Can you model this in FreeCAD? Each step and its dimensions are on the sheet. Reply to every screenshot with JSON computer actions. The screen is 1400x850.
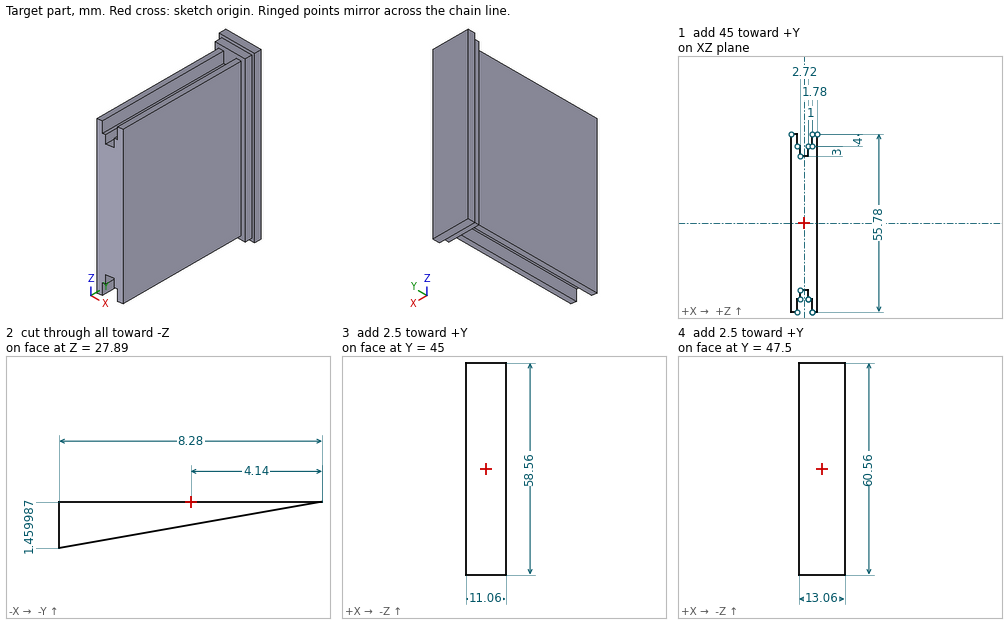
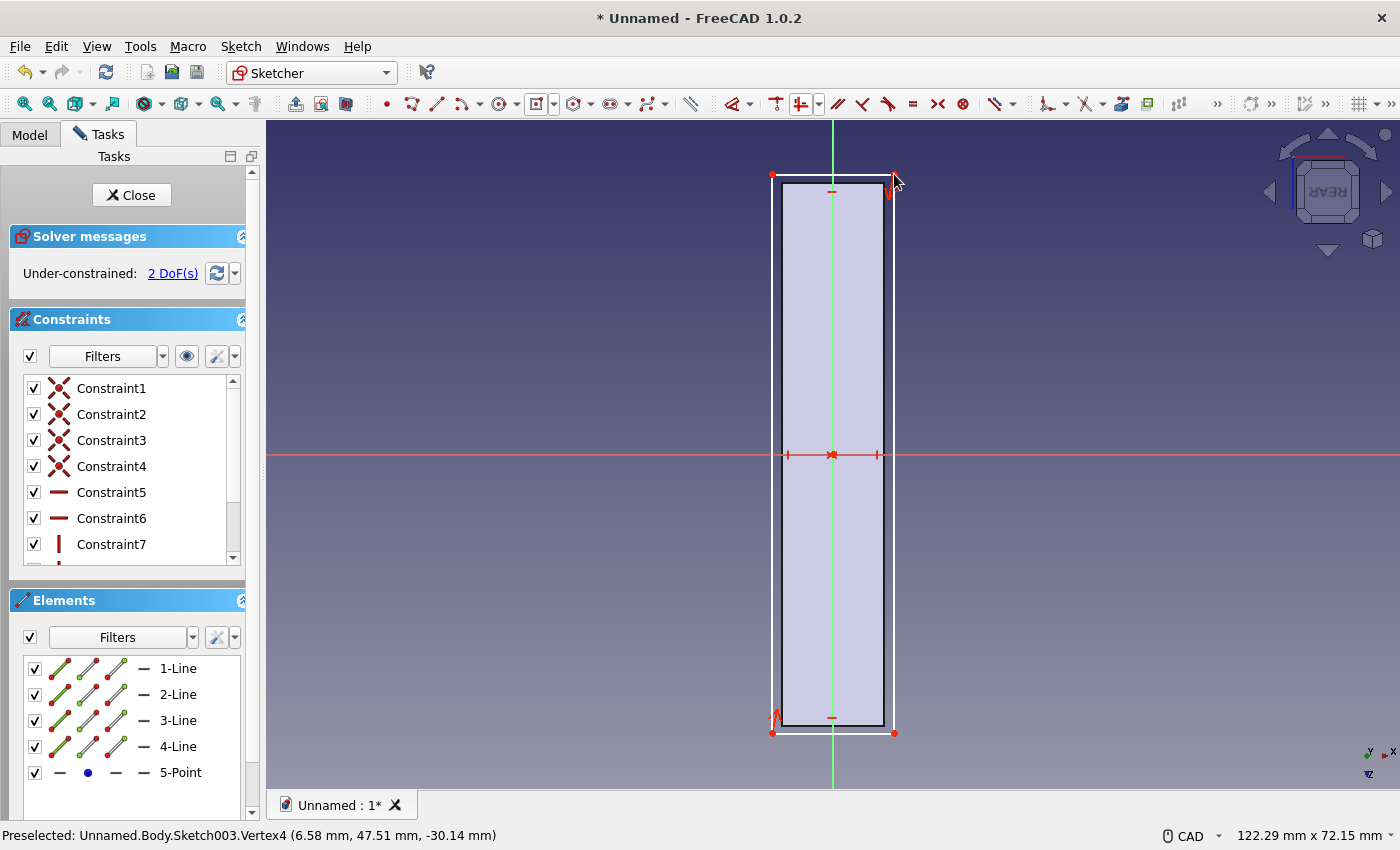
{"action": "left_click", "coordinate": [732, 104]}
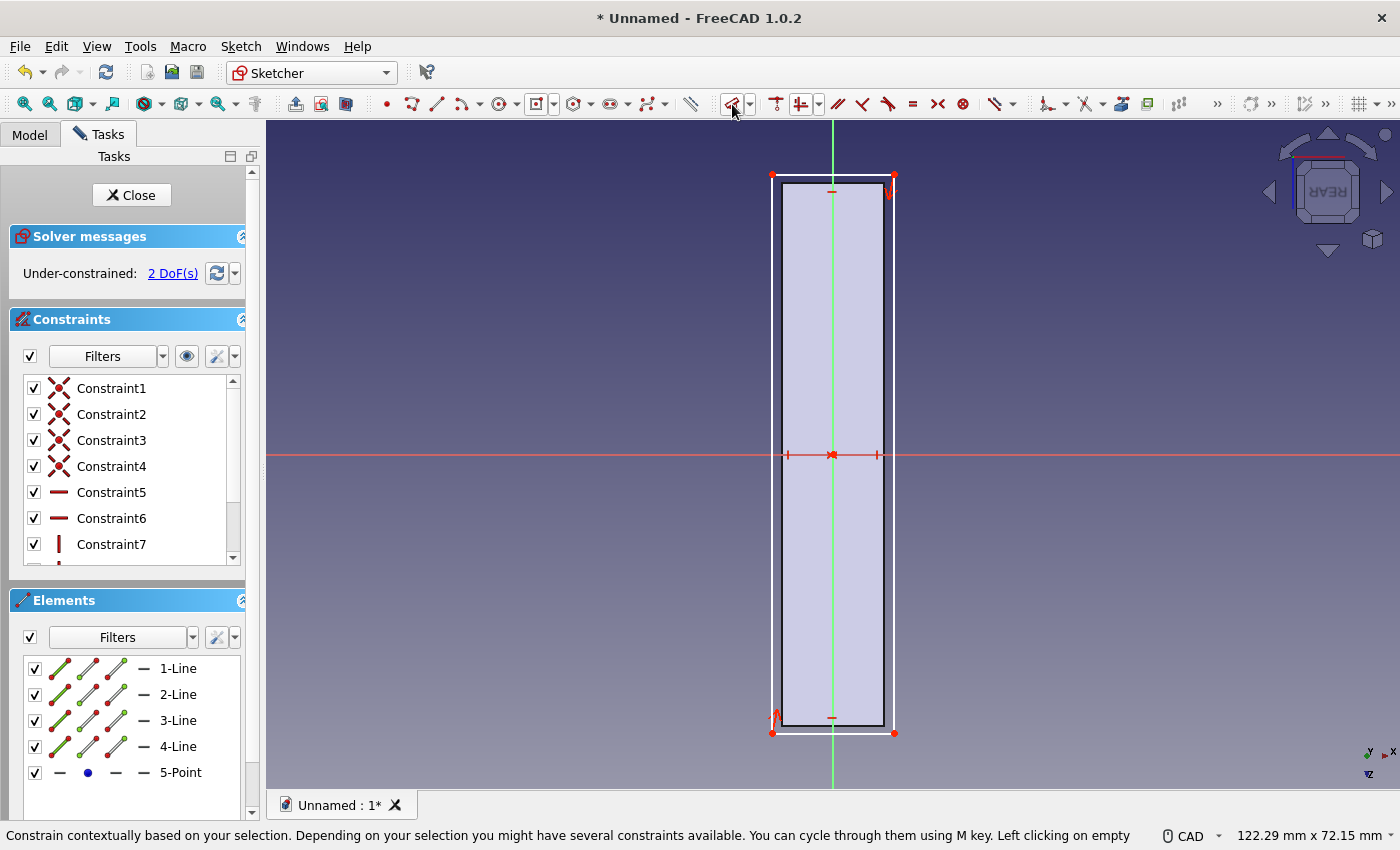
{"action": "left_click", "coordinate": [809, 734]}
{"action": "left_click", "coordinate": [805, 700]}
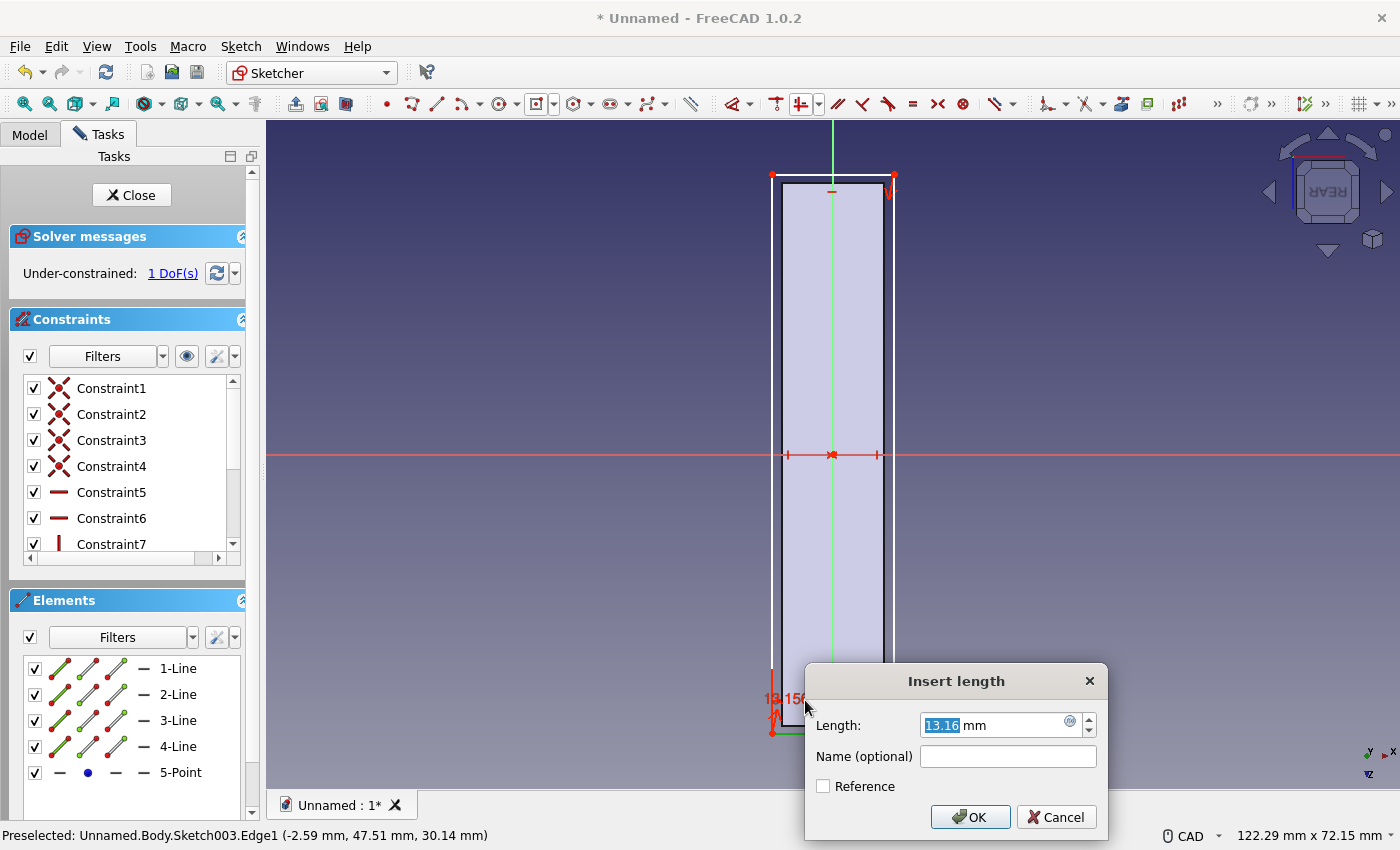
{"action": "type", "text": "13.06"}
{"action": "key", "text": "Return"}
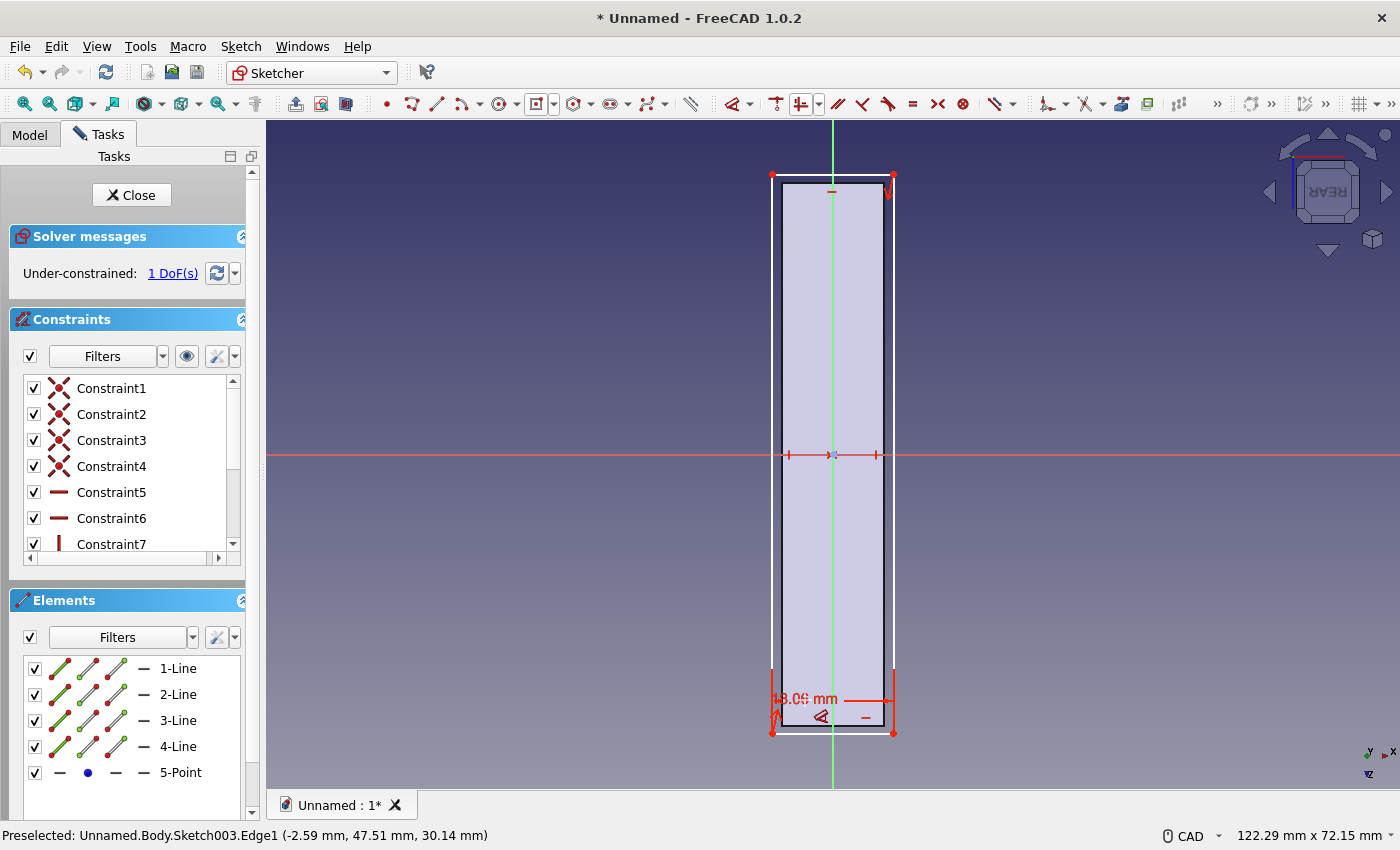
{"action": "left_click", "coordinate": [894, 566]}
{"action": "left_click", "coordinate": [928, 326]}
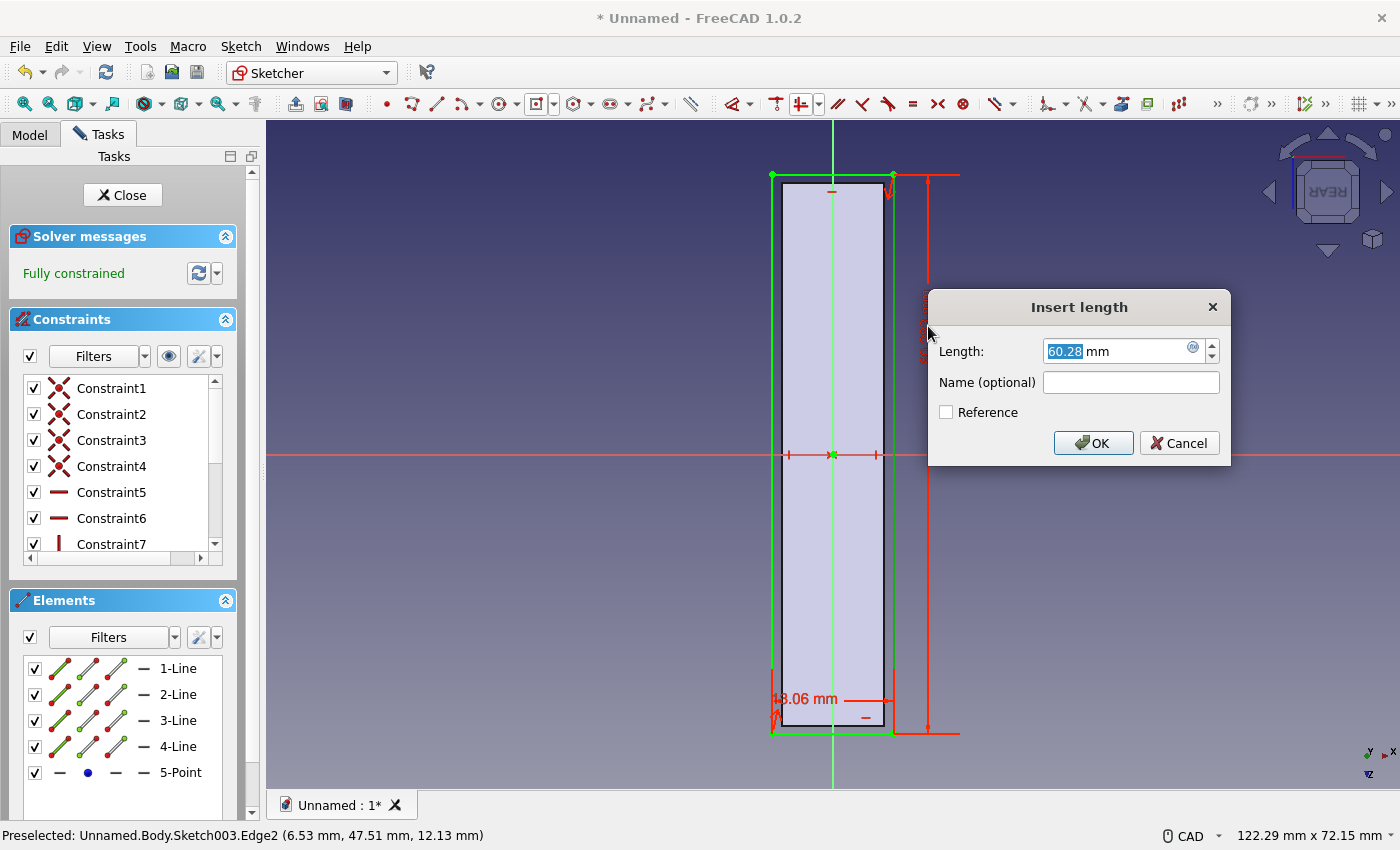
{"action": "type", "text": "60.56"}
{"action": "key", "text": "Return"}
{"action": "key", "text": "Escape"}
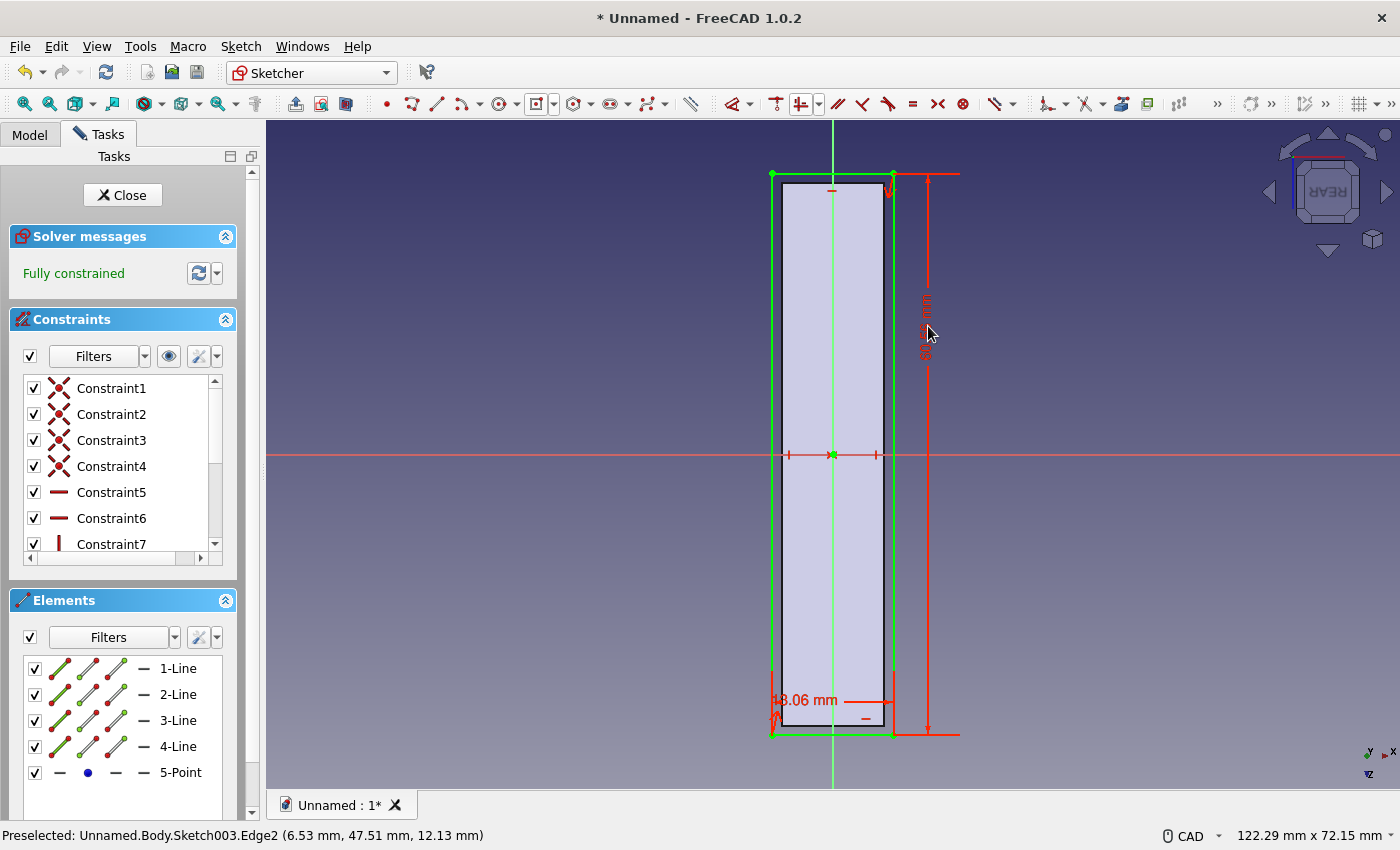
{"action": "left_click", "coordinate": [123, 195]}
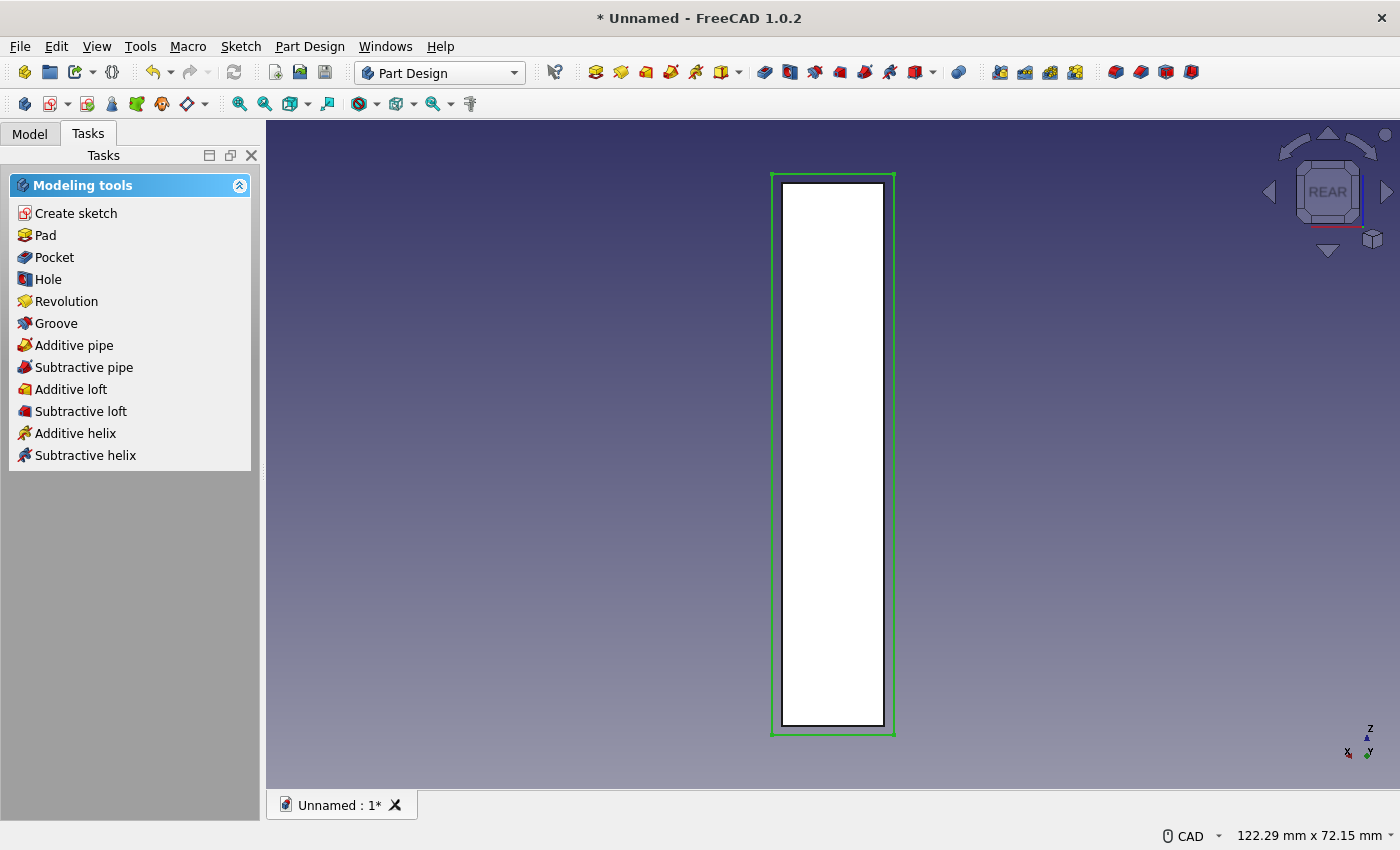
{"action": "left_click", "coordinate": [596, 72]}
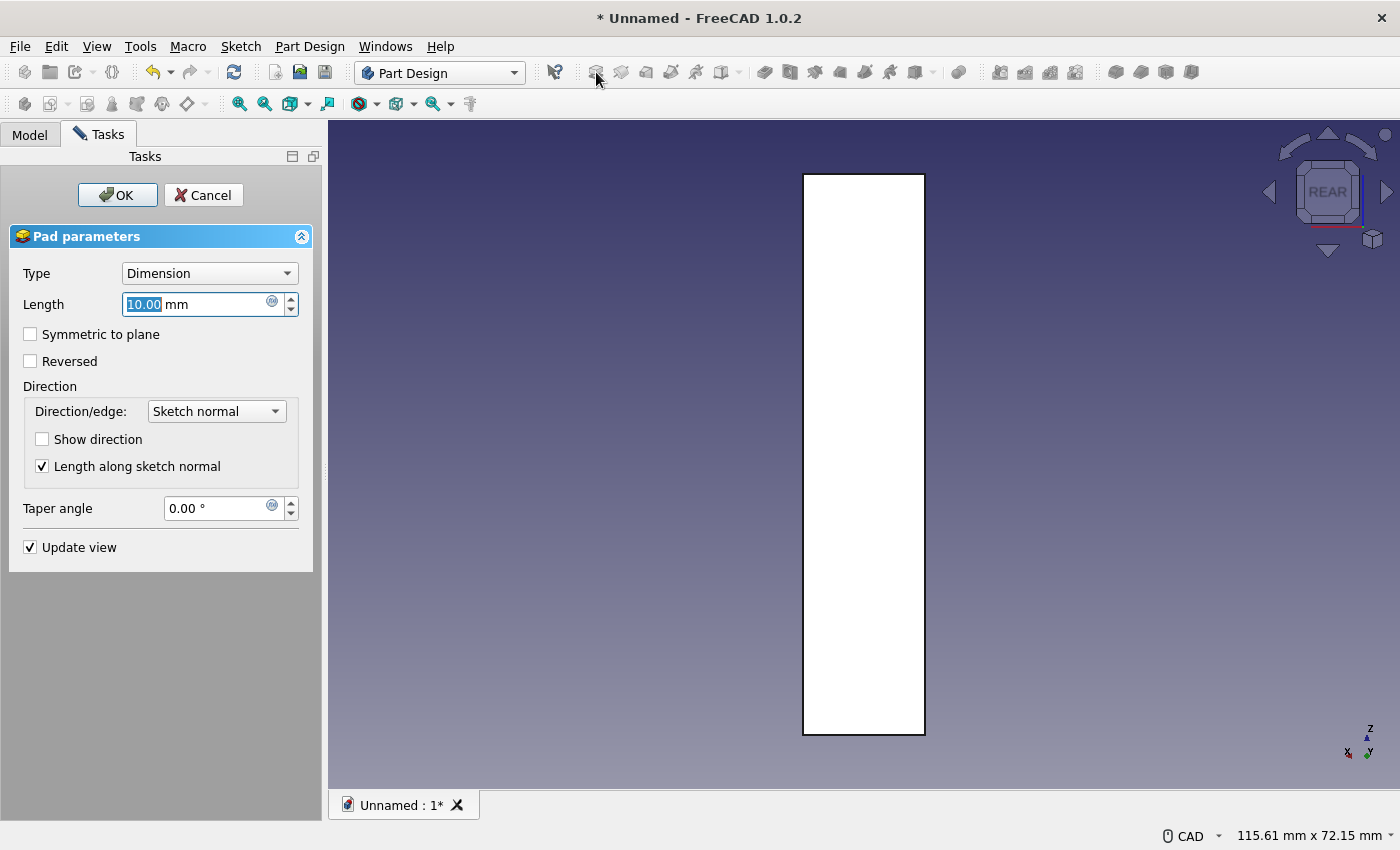
{"action": "type", "text": "2.5"}
{"action": "key", "text": "Tab"}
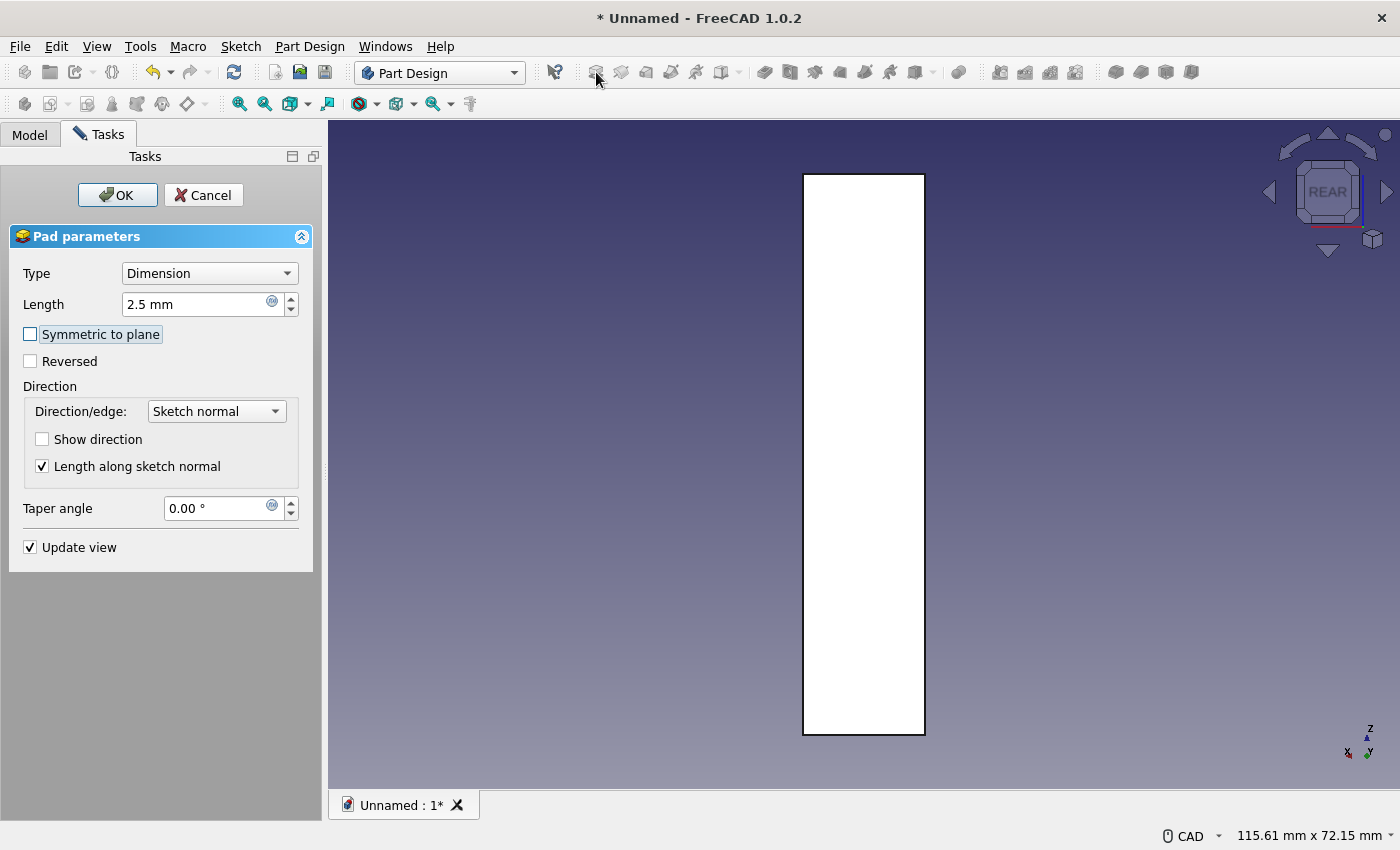
{"action": "left_click", "coordinate": [118, 195]}